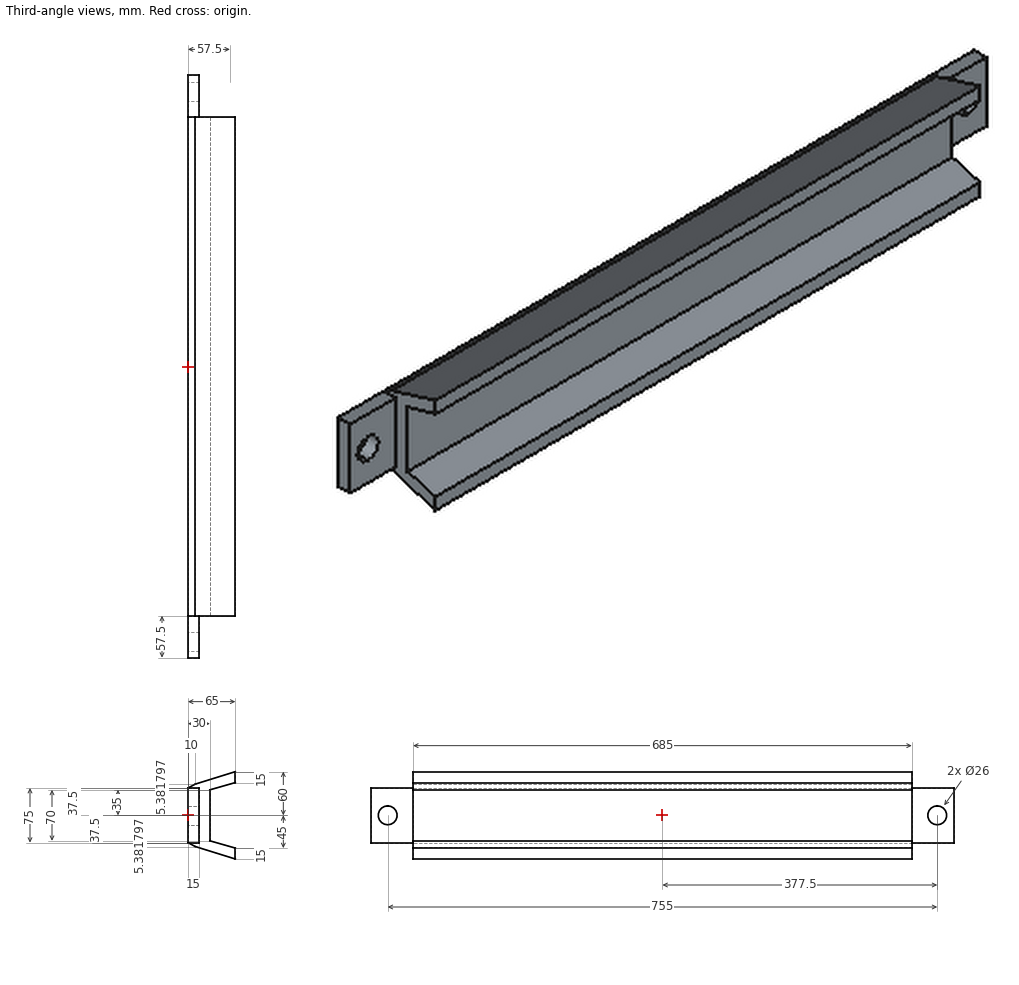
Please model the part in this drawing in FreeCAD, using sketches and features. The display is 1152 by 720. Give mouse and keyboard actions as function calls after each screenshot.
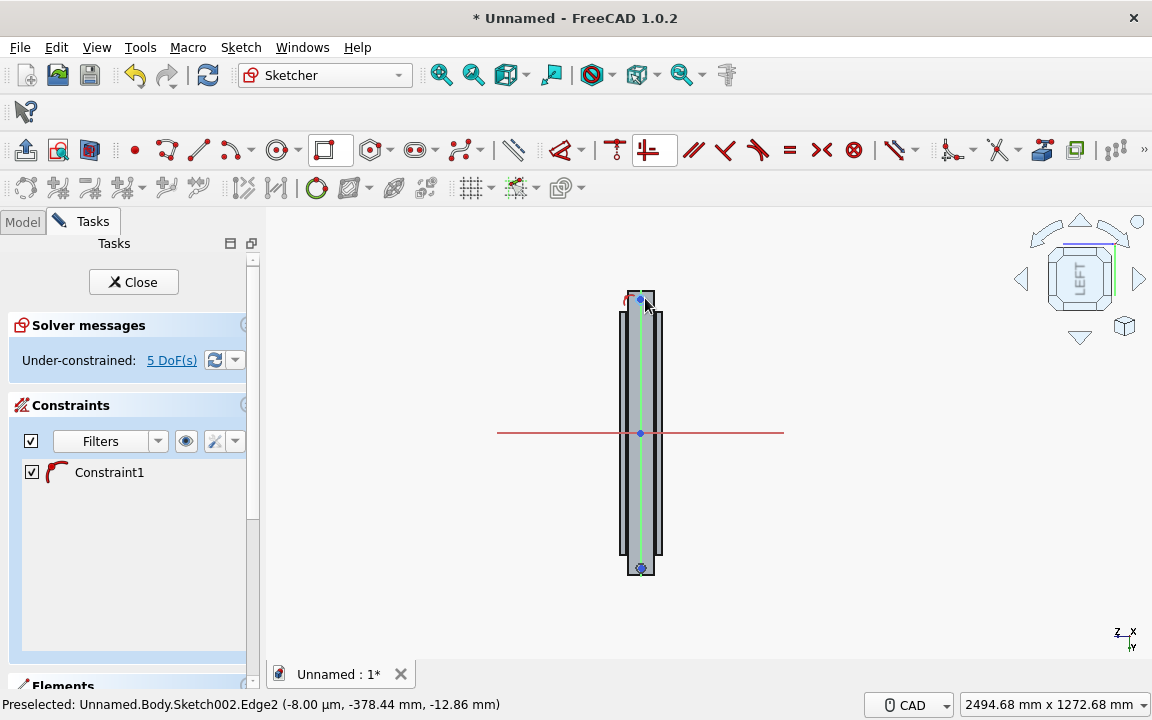
scroll(644, 565, up, 8)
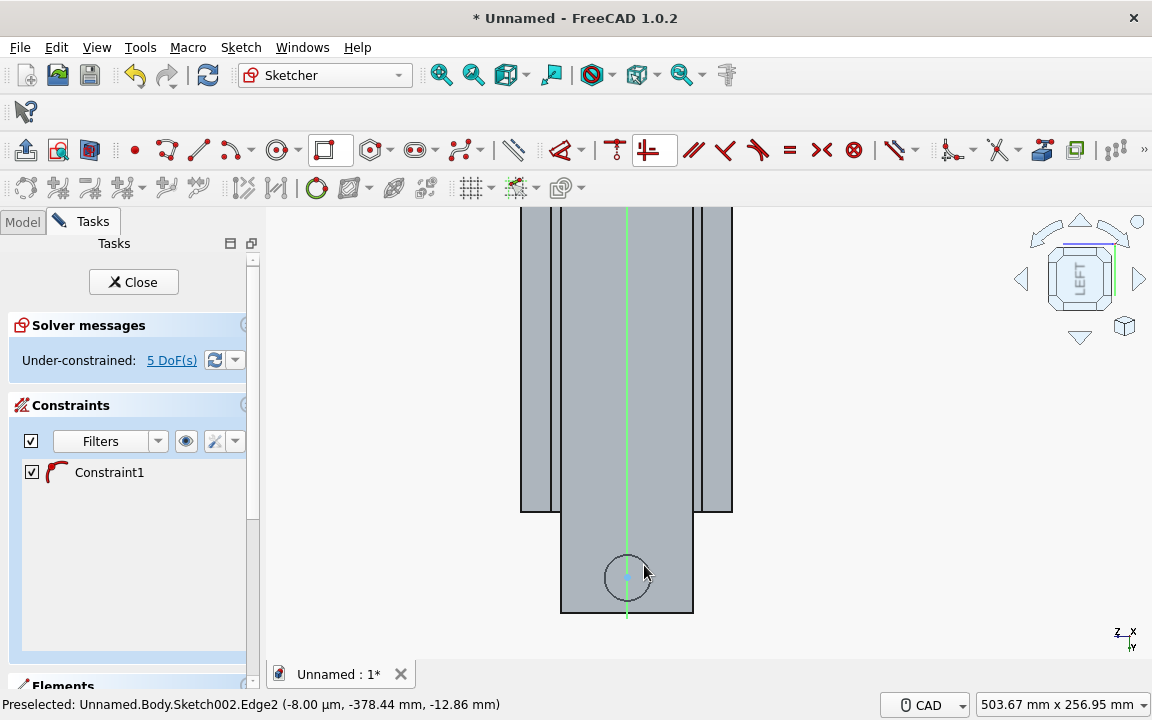
click(644, 562)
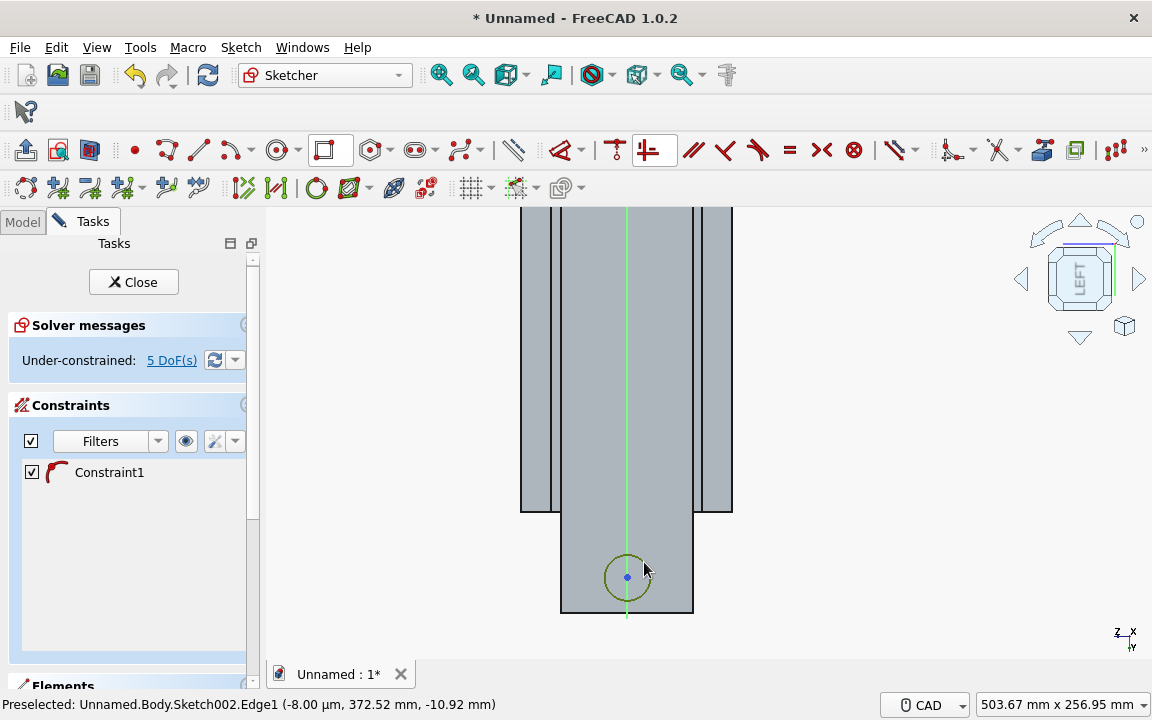
scroll(644, 566, down, 8)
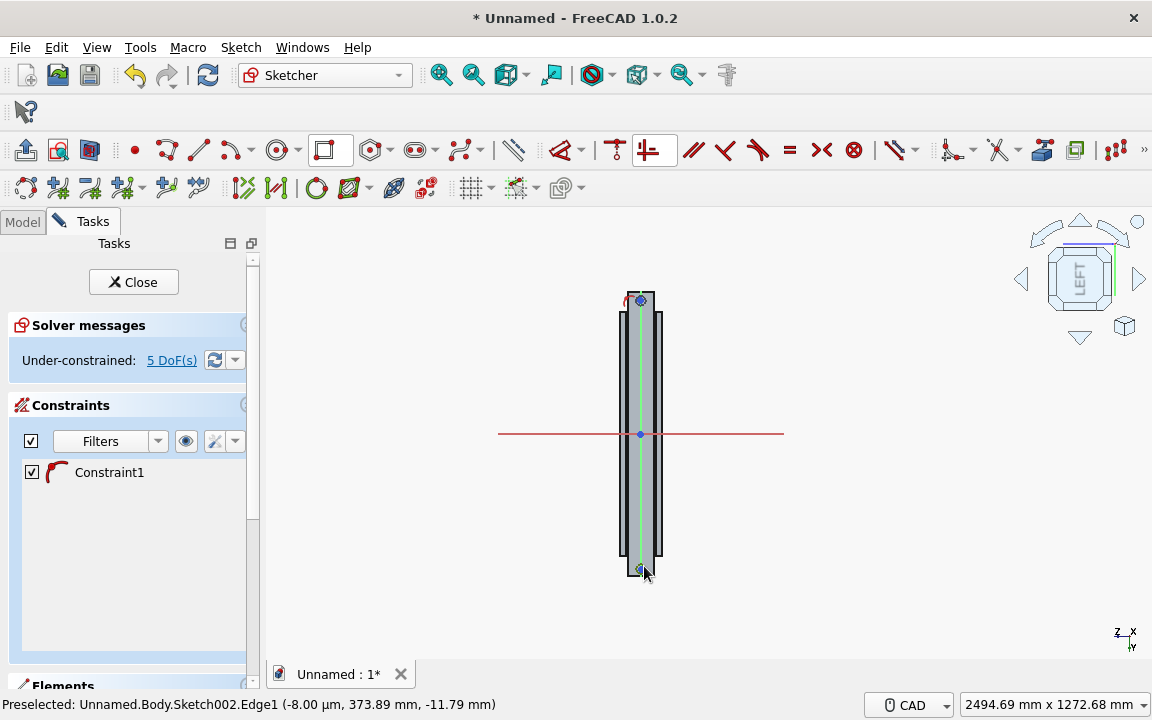
scroll(644, 297, up, 8)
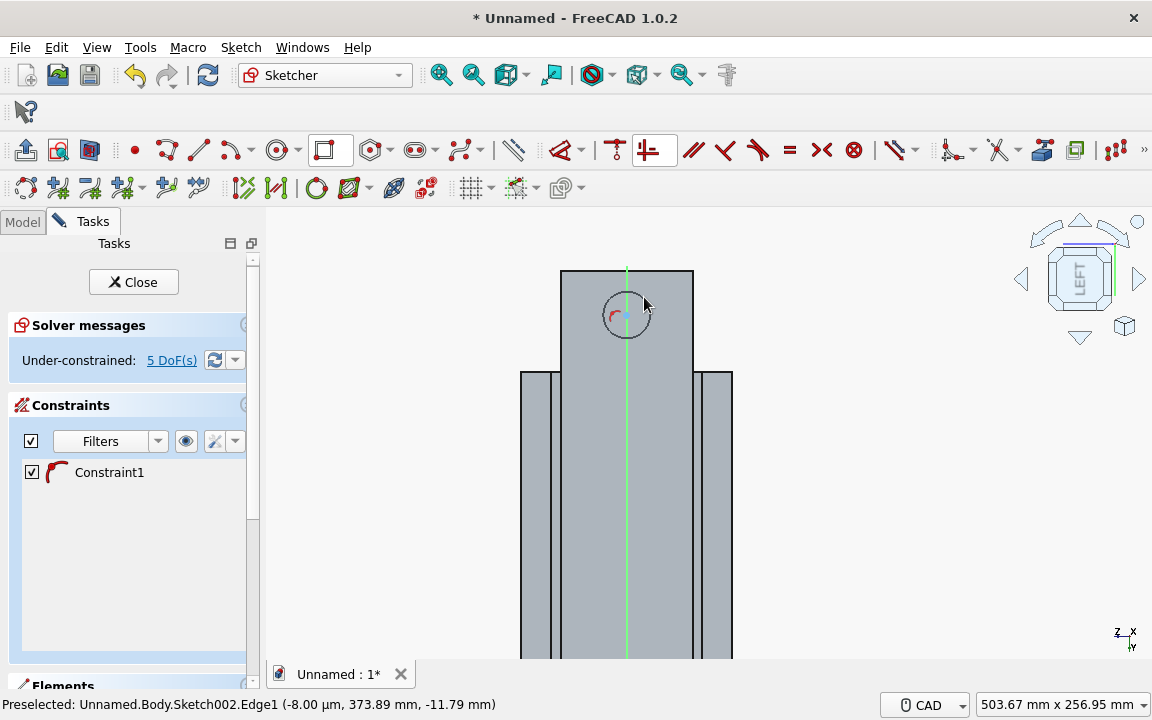
click(643, 298)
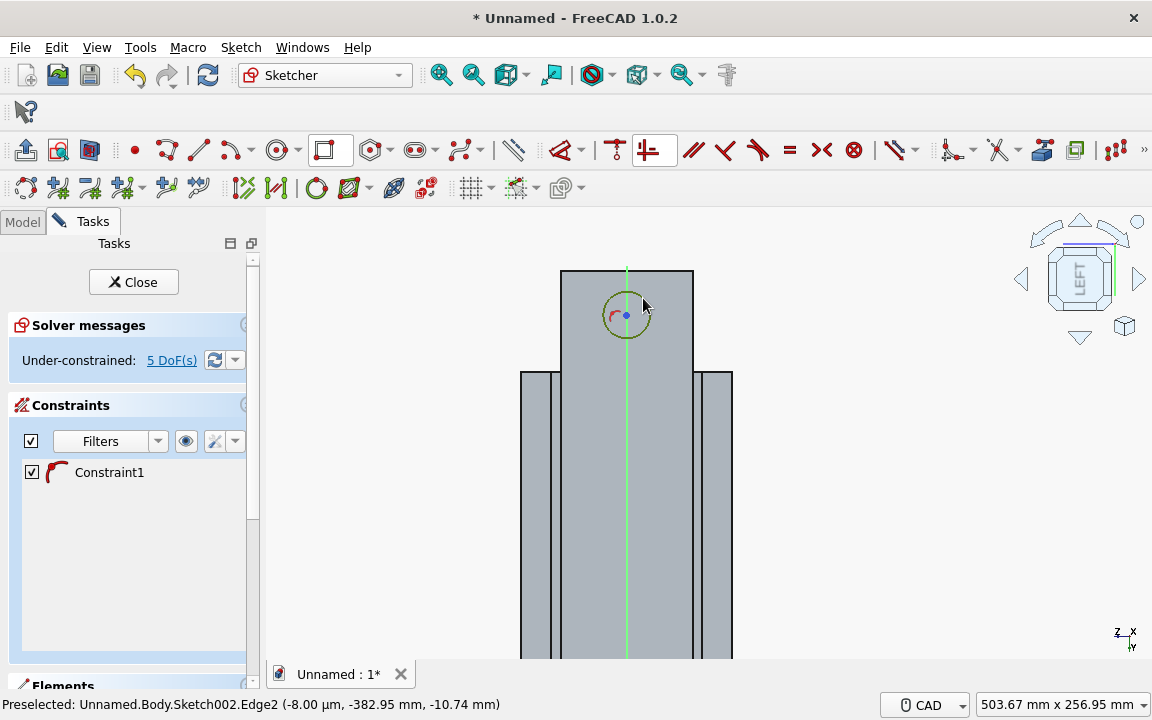
click(790, 150)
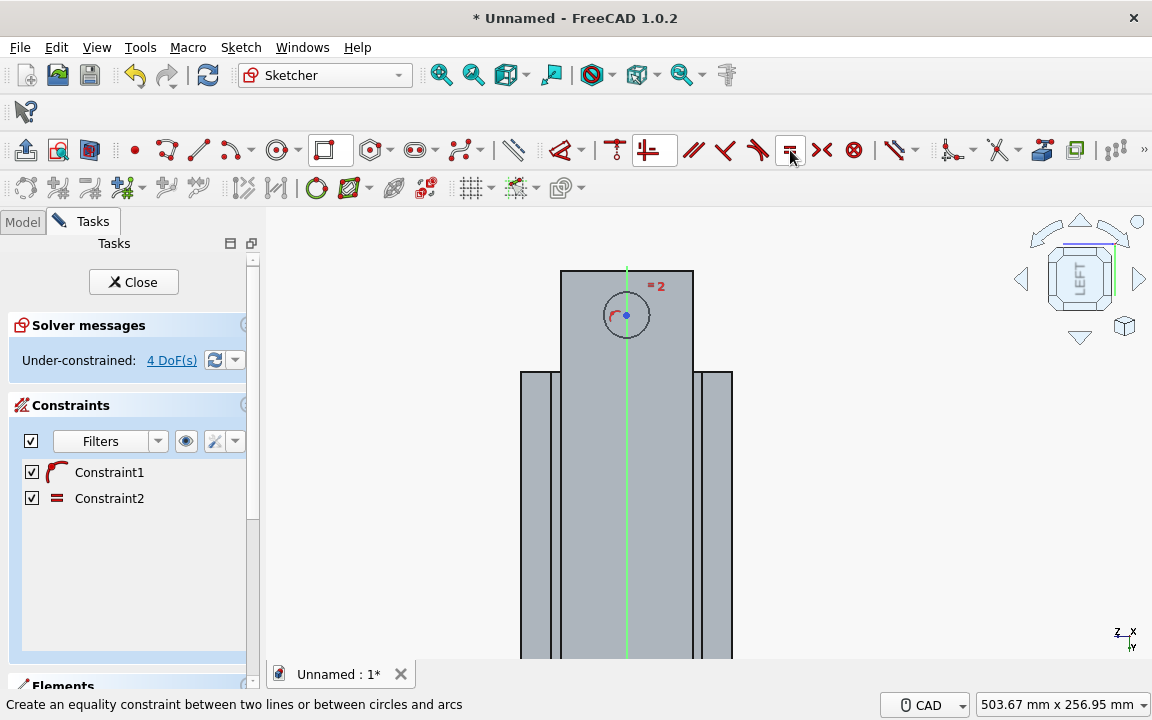
scroll(644, 296, down, 8)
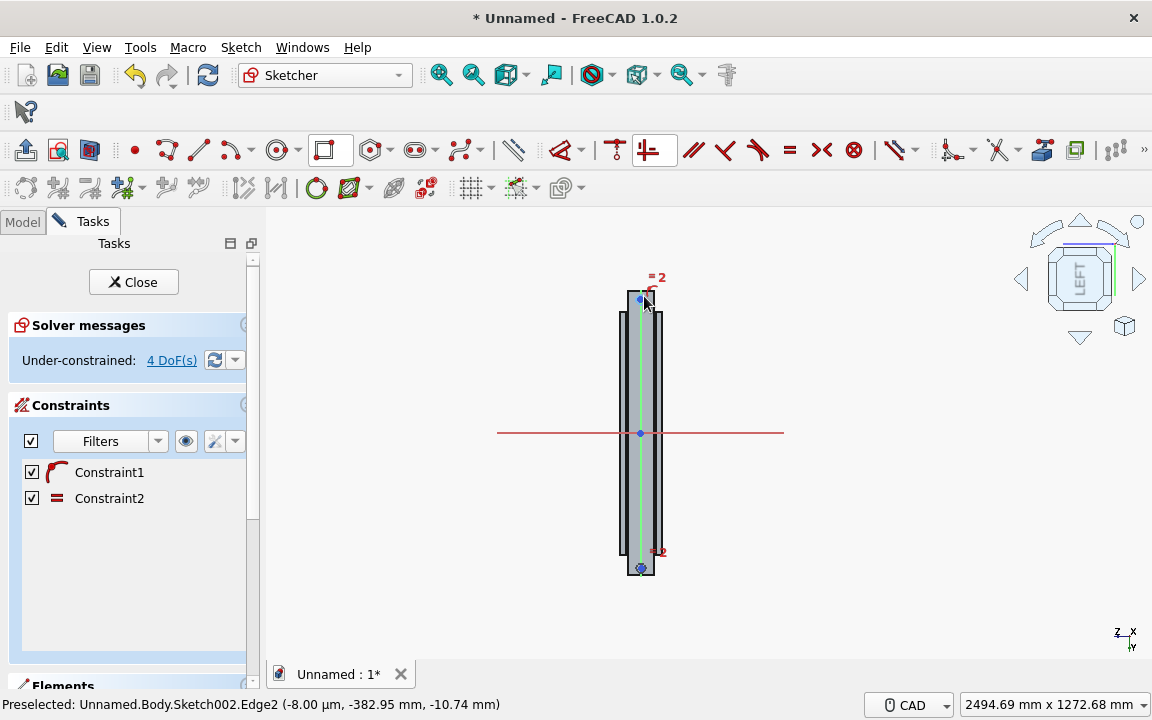
click(641, 568)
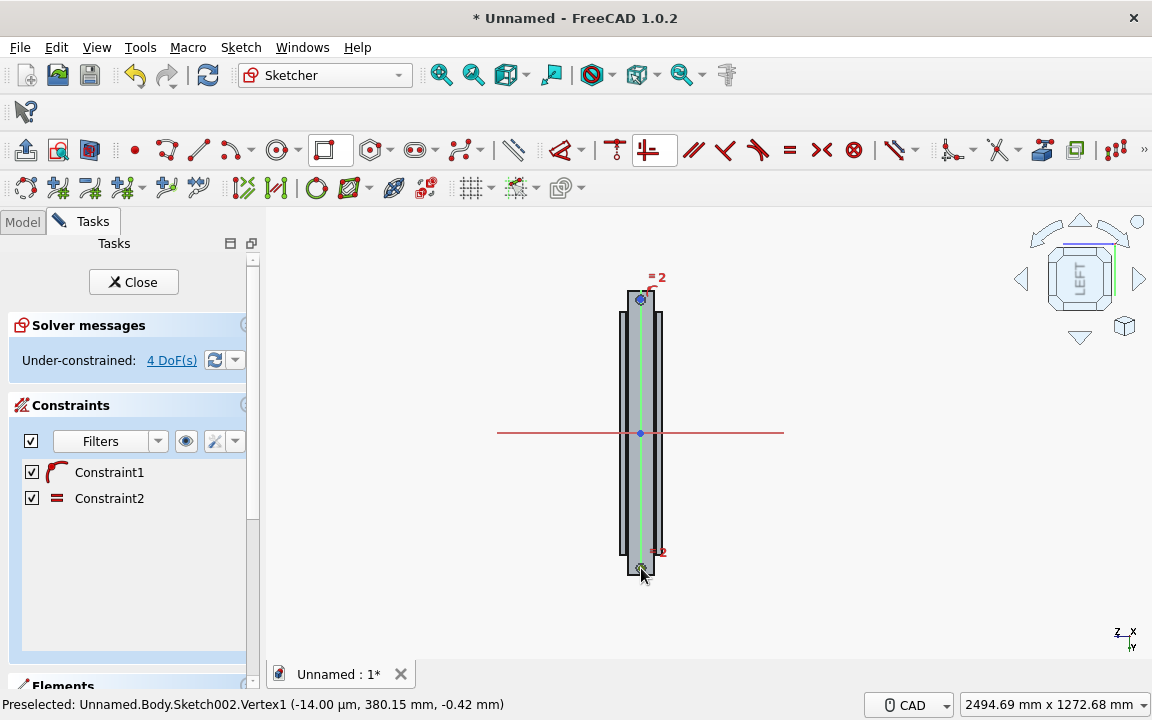
click(641, 518)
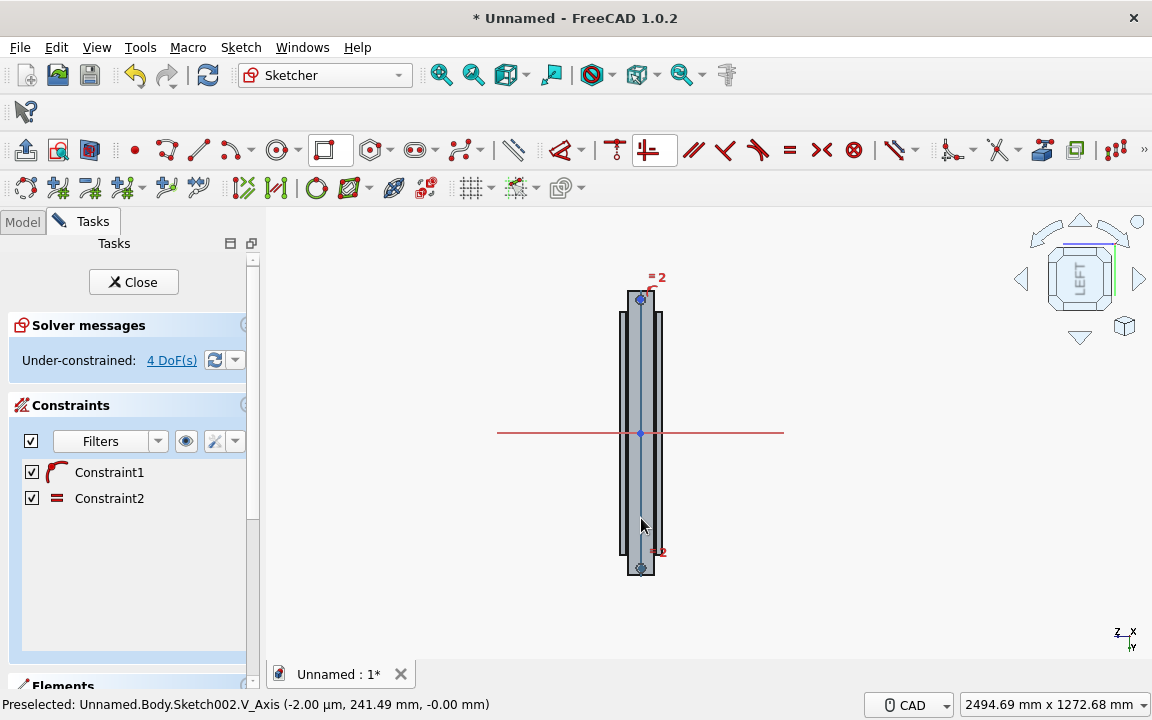
click(616, 150)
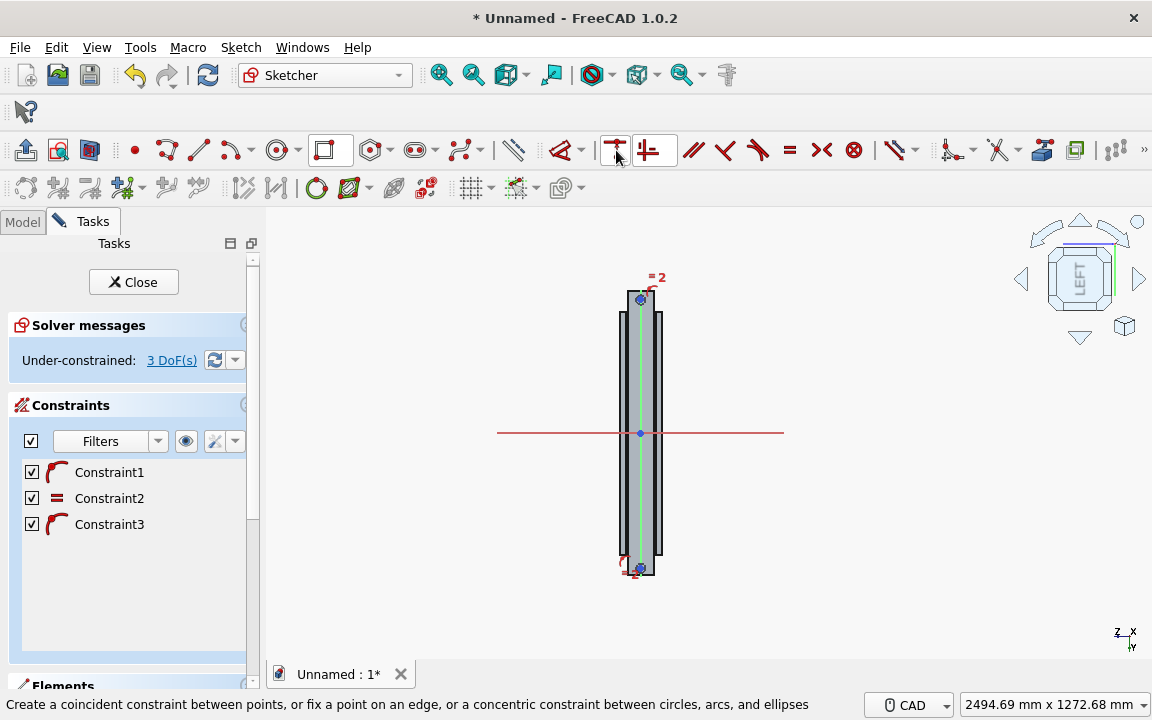
click(560, 150)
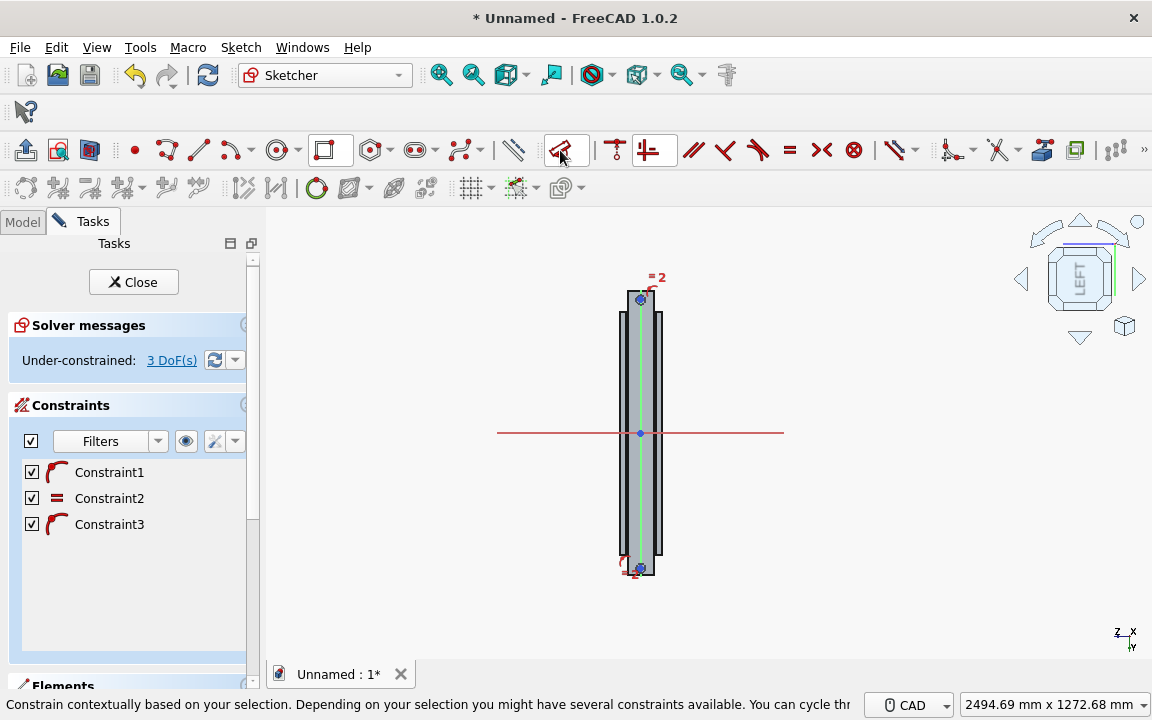
scroll(641, 564, up, 8)